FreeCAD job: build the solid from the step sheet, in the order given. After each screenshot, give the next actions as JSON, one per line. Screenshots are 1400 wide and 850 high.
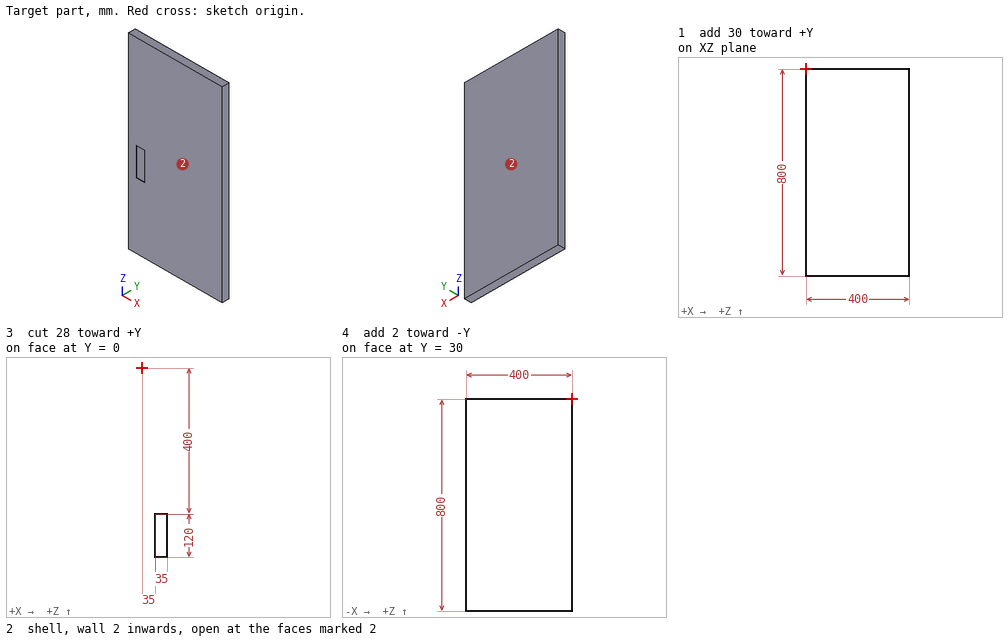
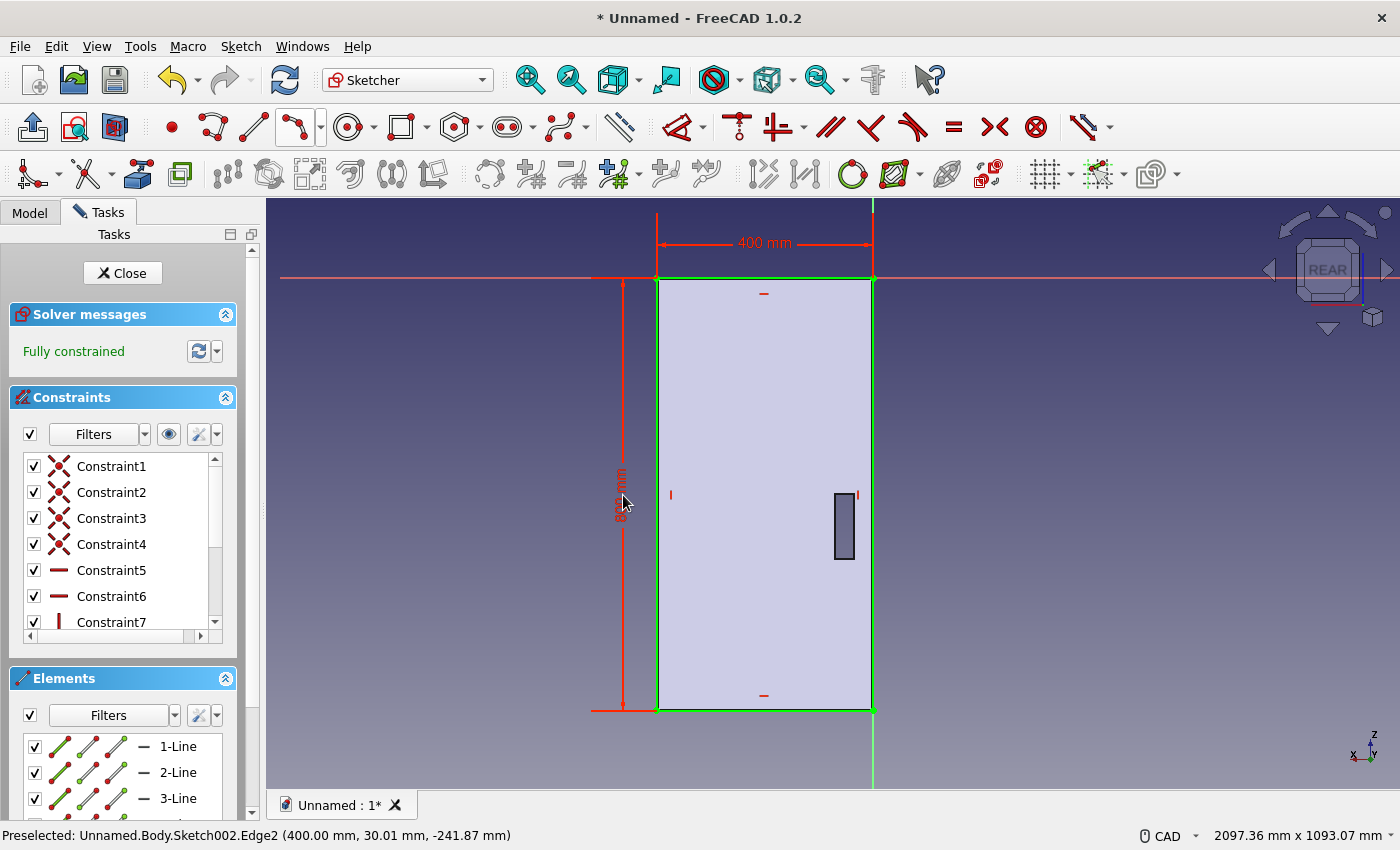
{"action": "left_click", "coordinate": [123, 273]}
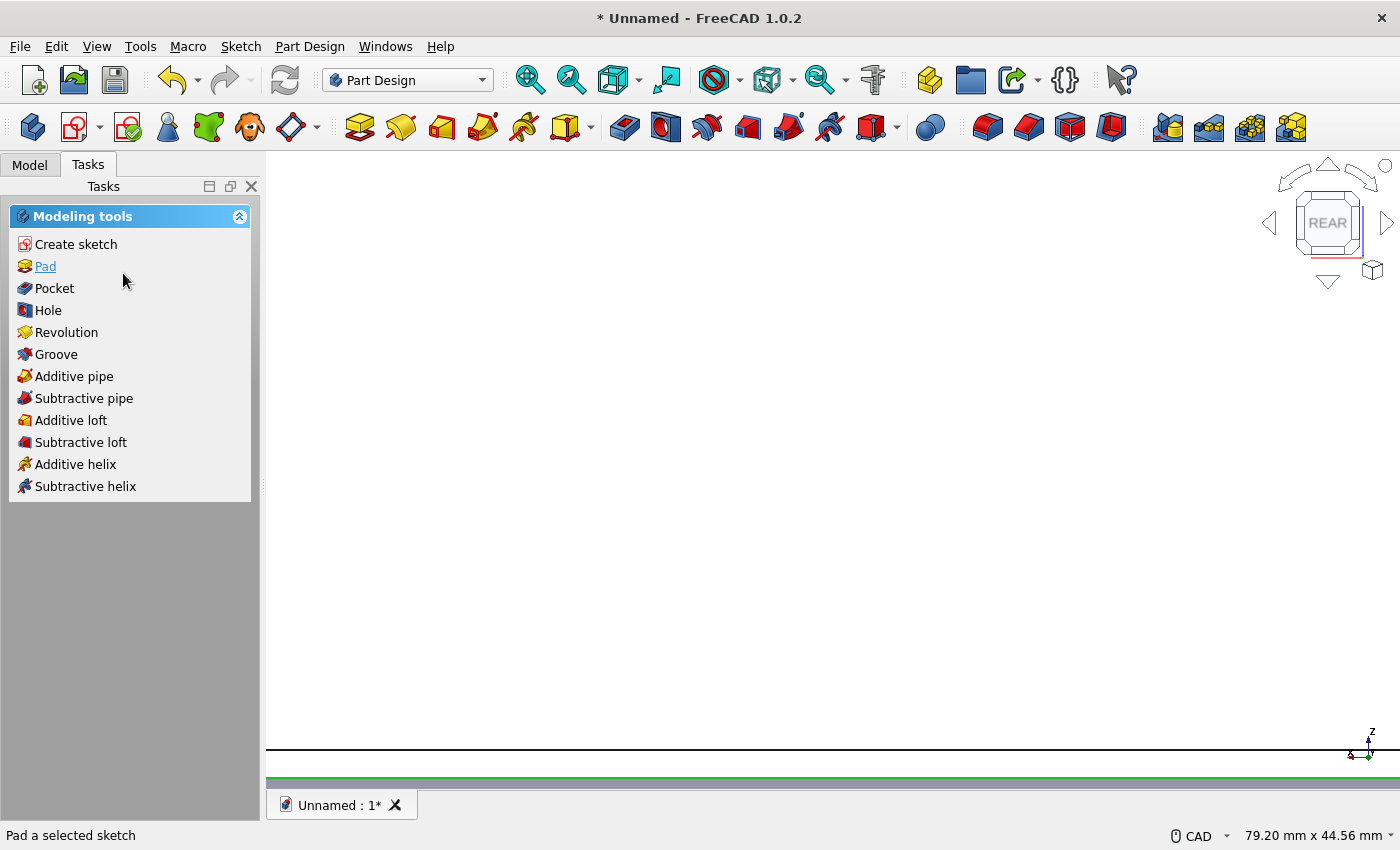
{"action": "left_click", "coordinate": [360, 128]}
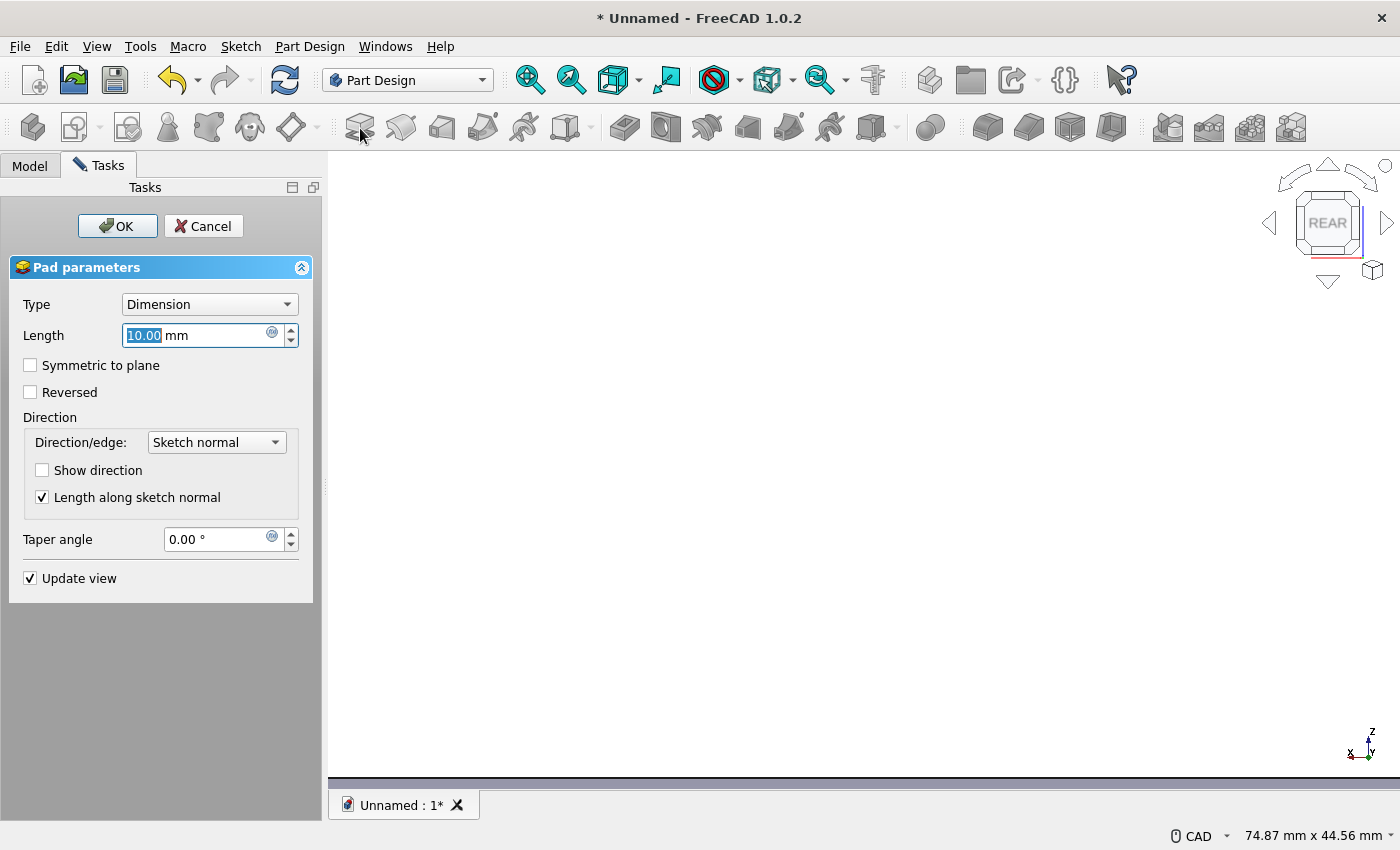
{"action": "type", "text": "2"}
{"action": "key", "text": "Tab"}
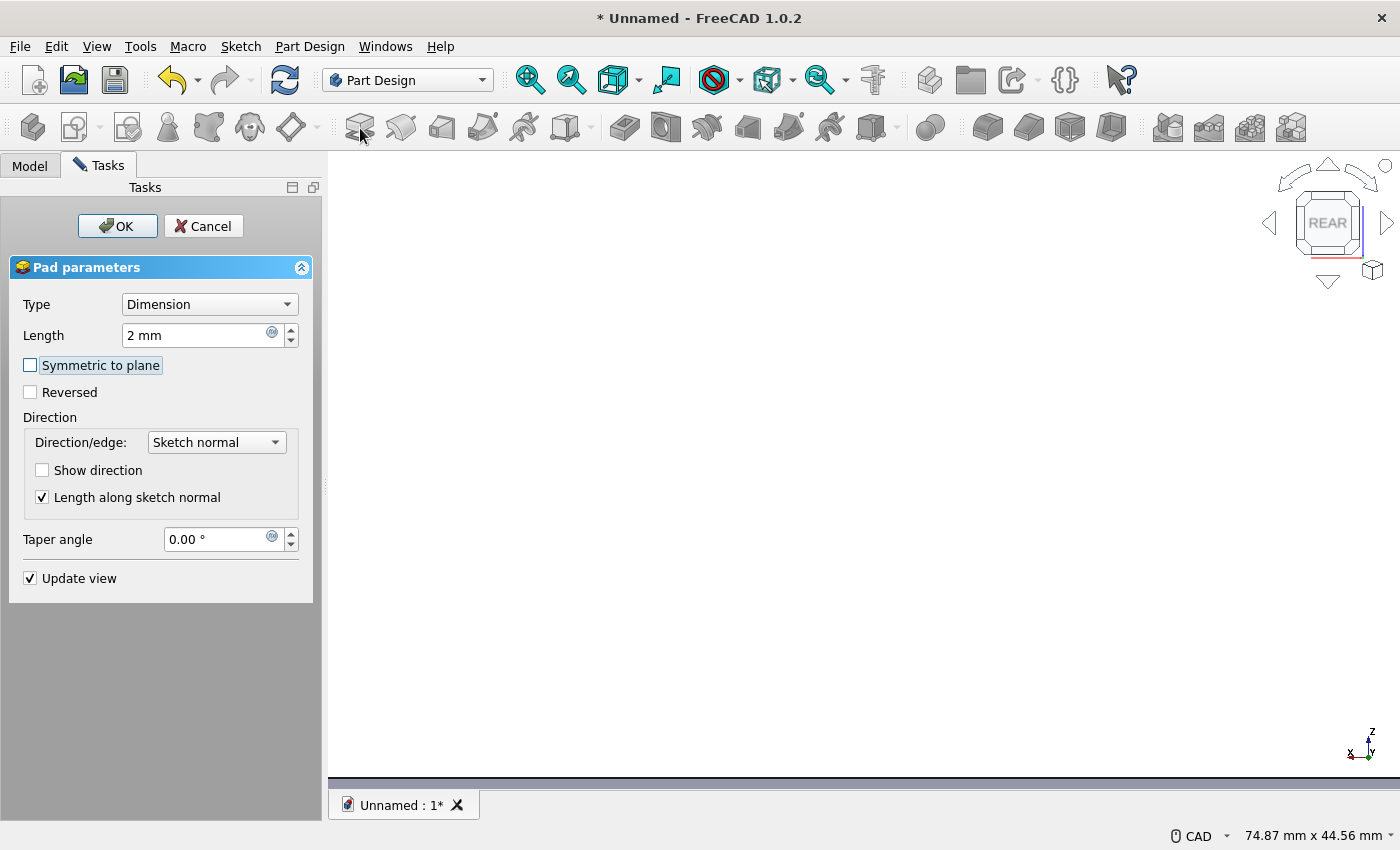
{"action": "left_click", "coordinate": [31, 392]}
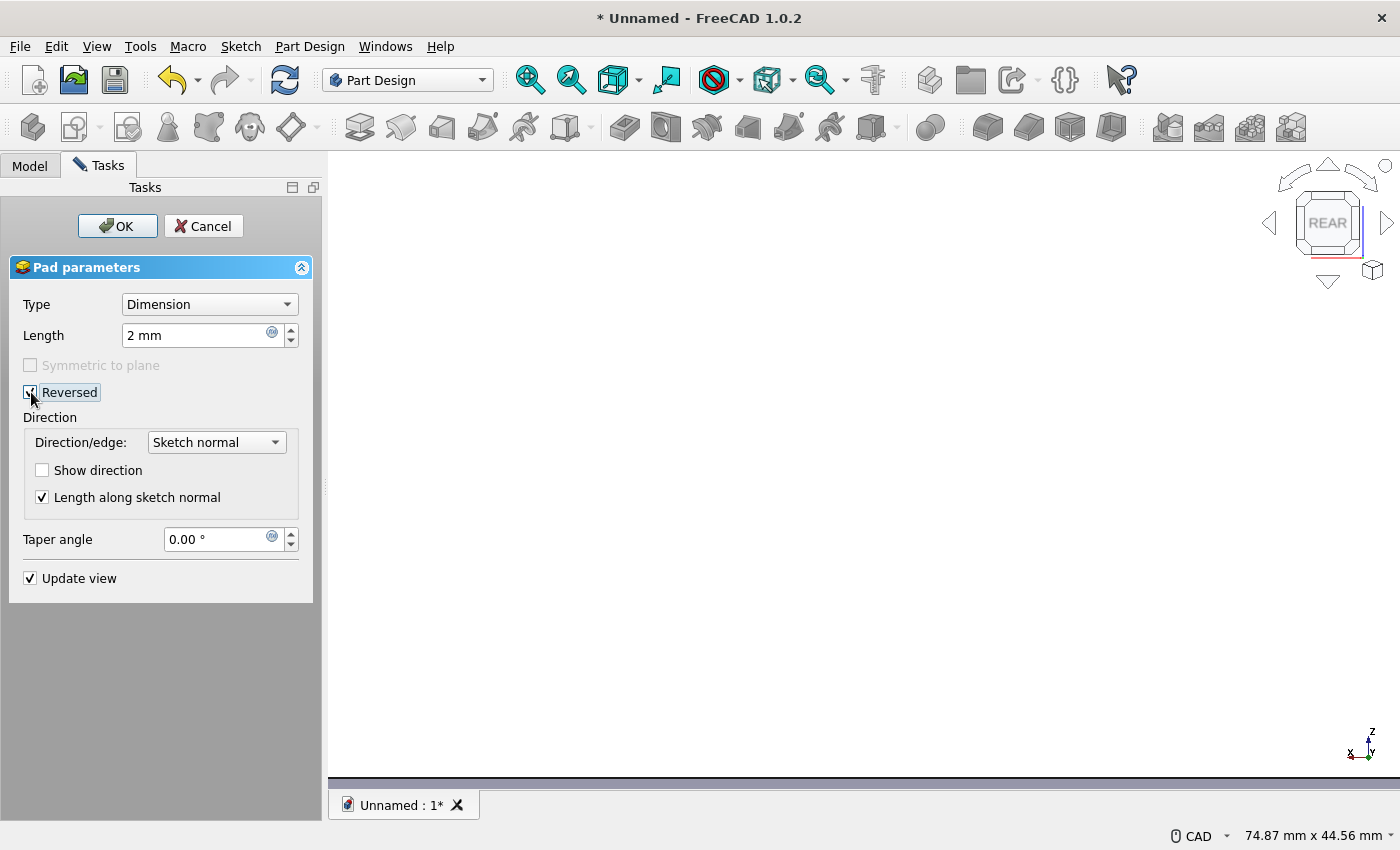
{"action": "left_click", "coordinate": [118, 226]}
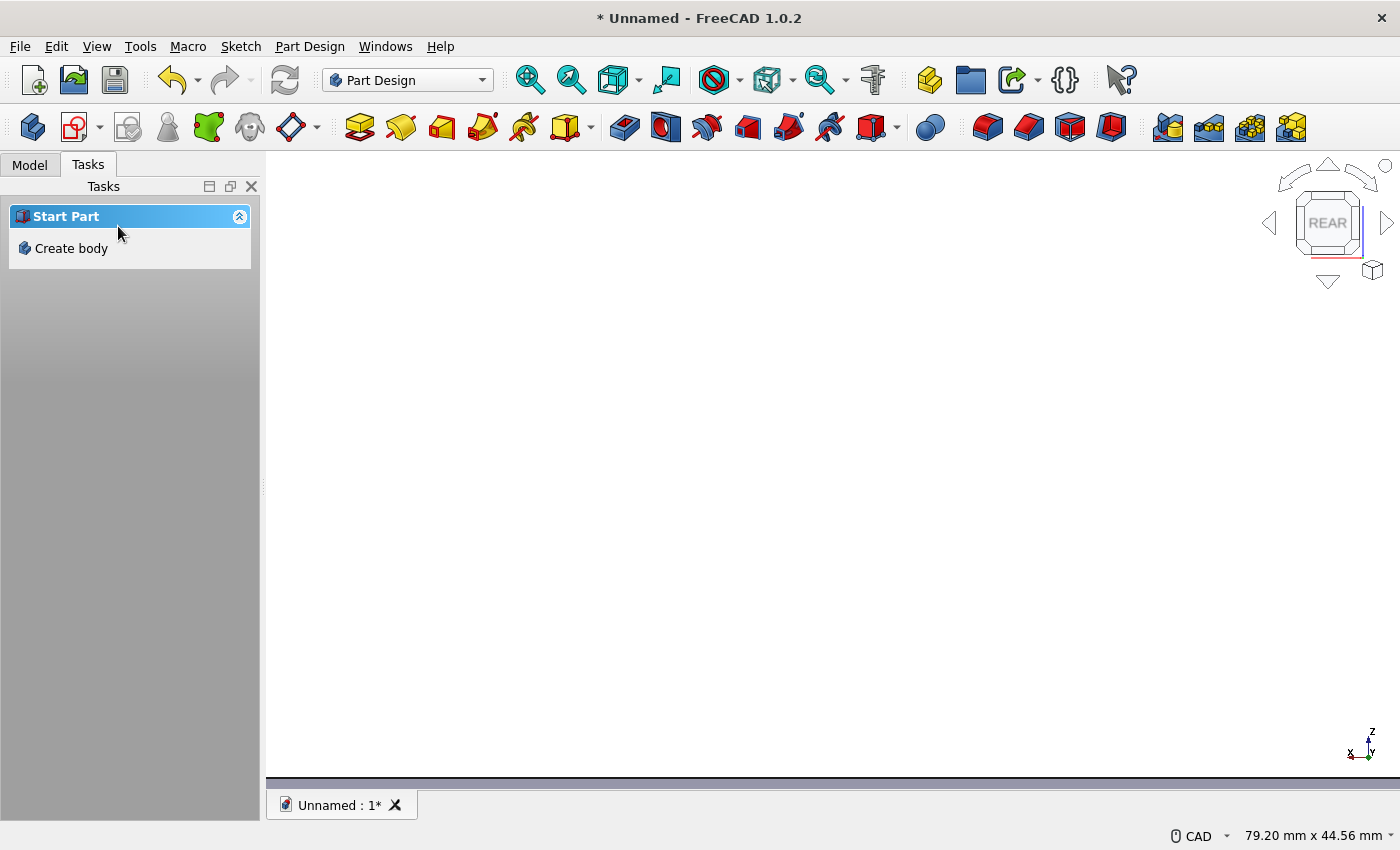
{"action": "key", "text": "0"}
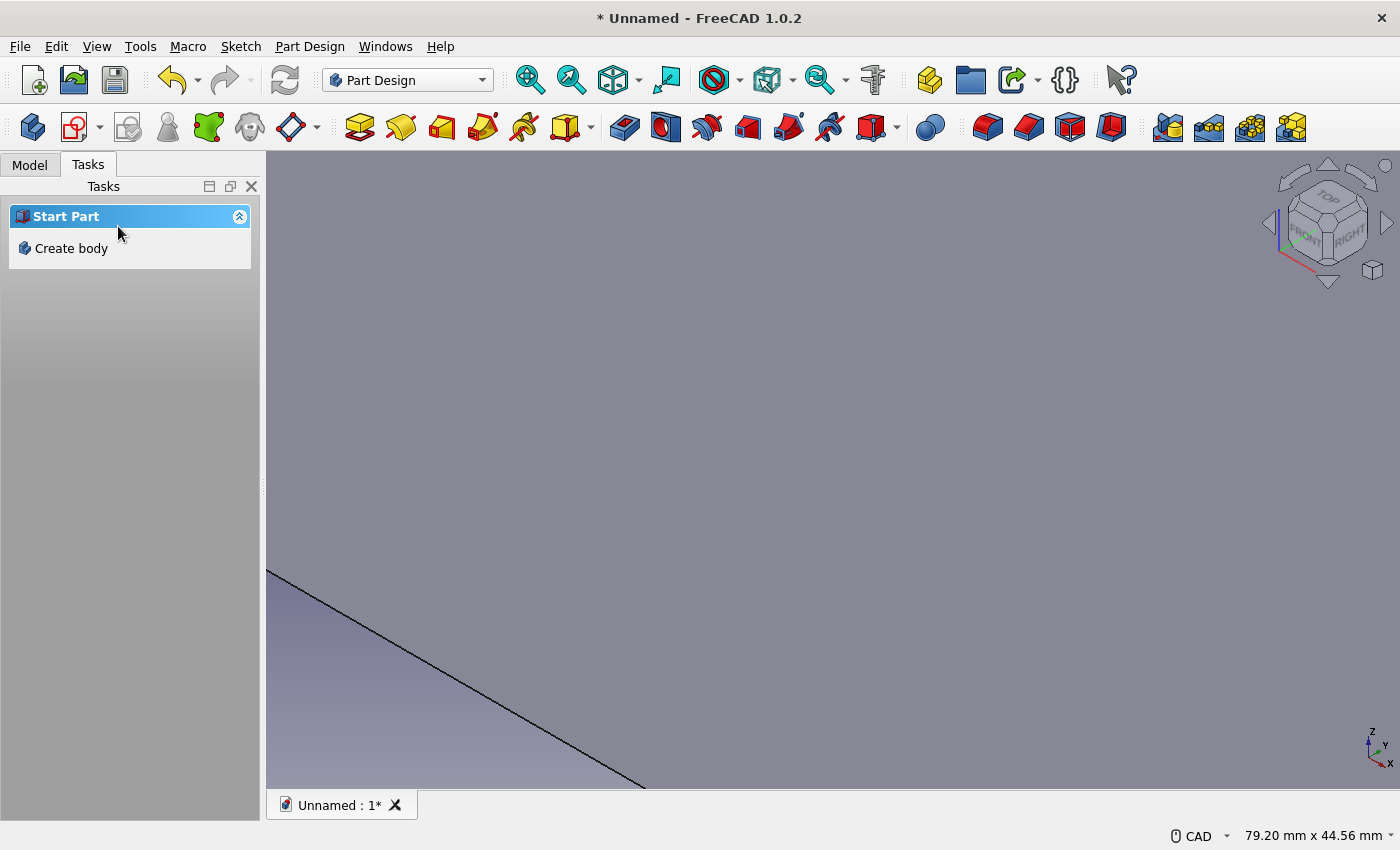
{"action": "left_click", "coordinate": [531, 80]}